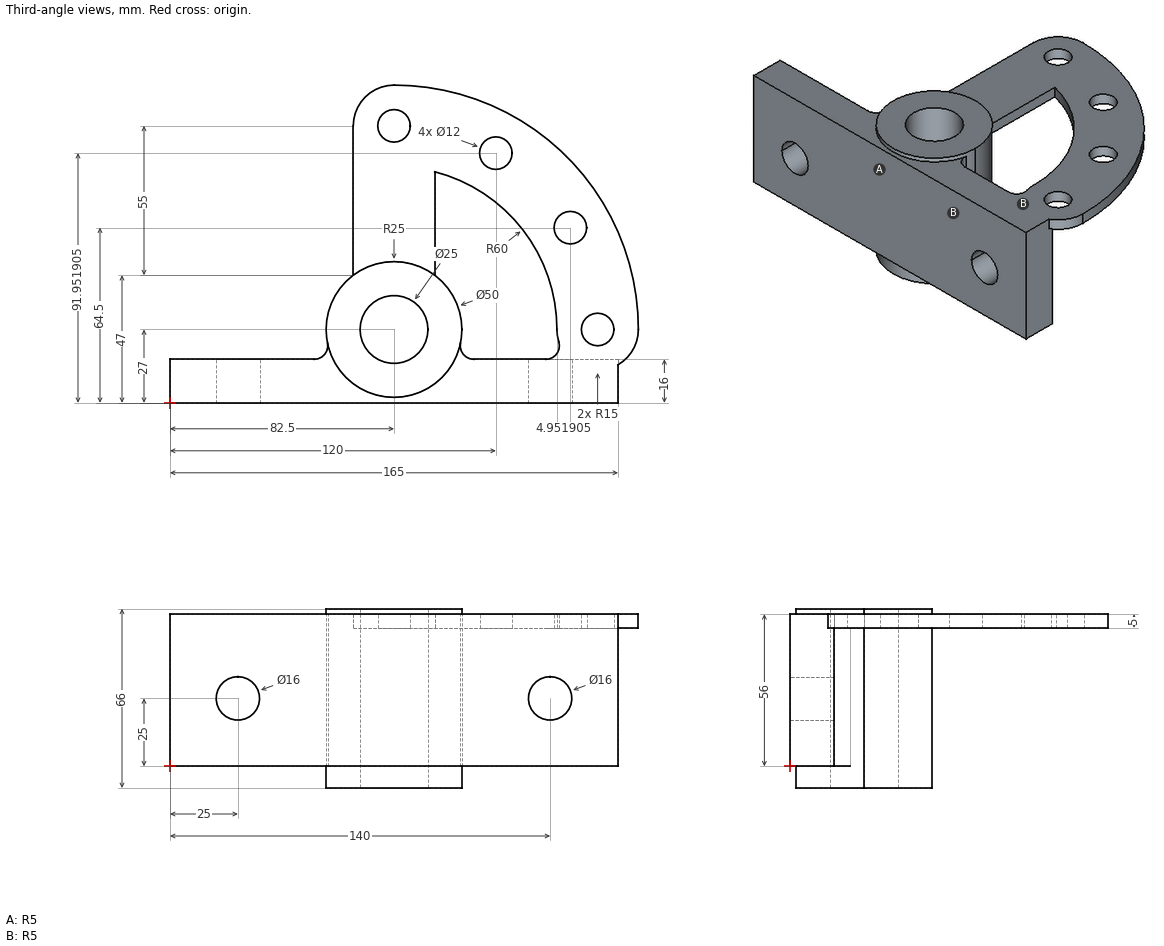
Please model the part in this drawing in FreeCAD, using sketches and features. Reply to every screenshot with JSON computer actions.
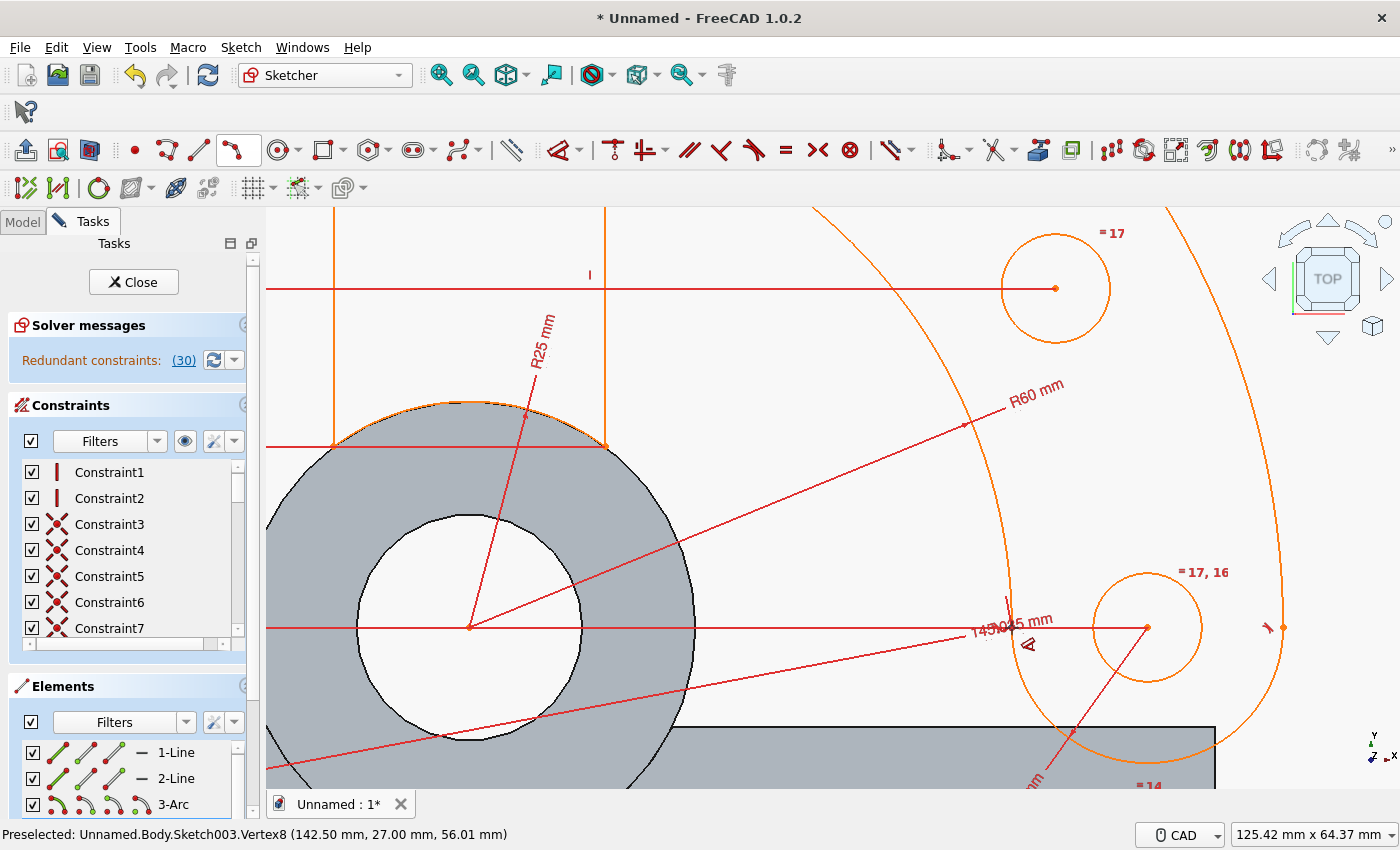
{"action": "left_click", "coordinate": [1056, 289]}
{"action": "left_click", "coordinate": [1034, 662]}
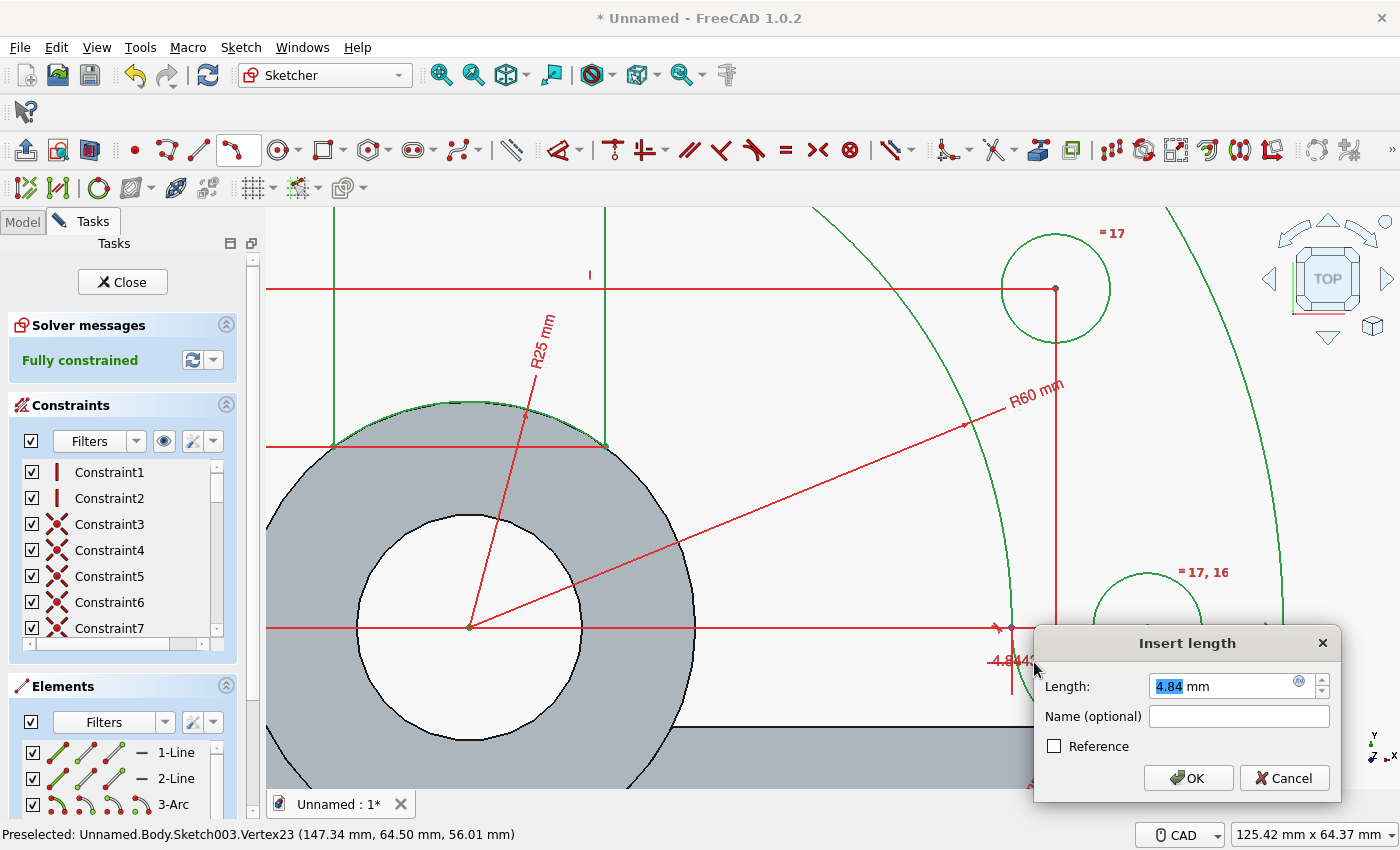
{"action": "type", "text": "4.951905"}
{"action": "key", "text": "Return"}
{"action": "key", "text": "Escape"}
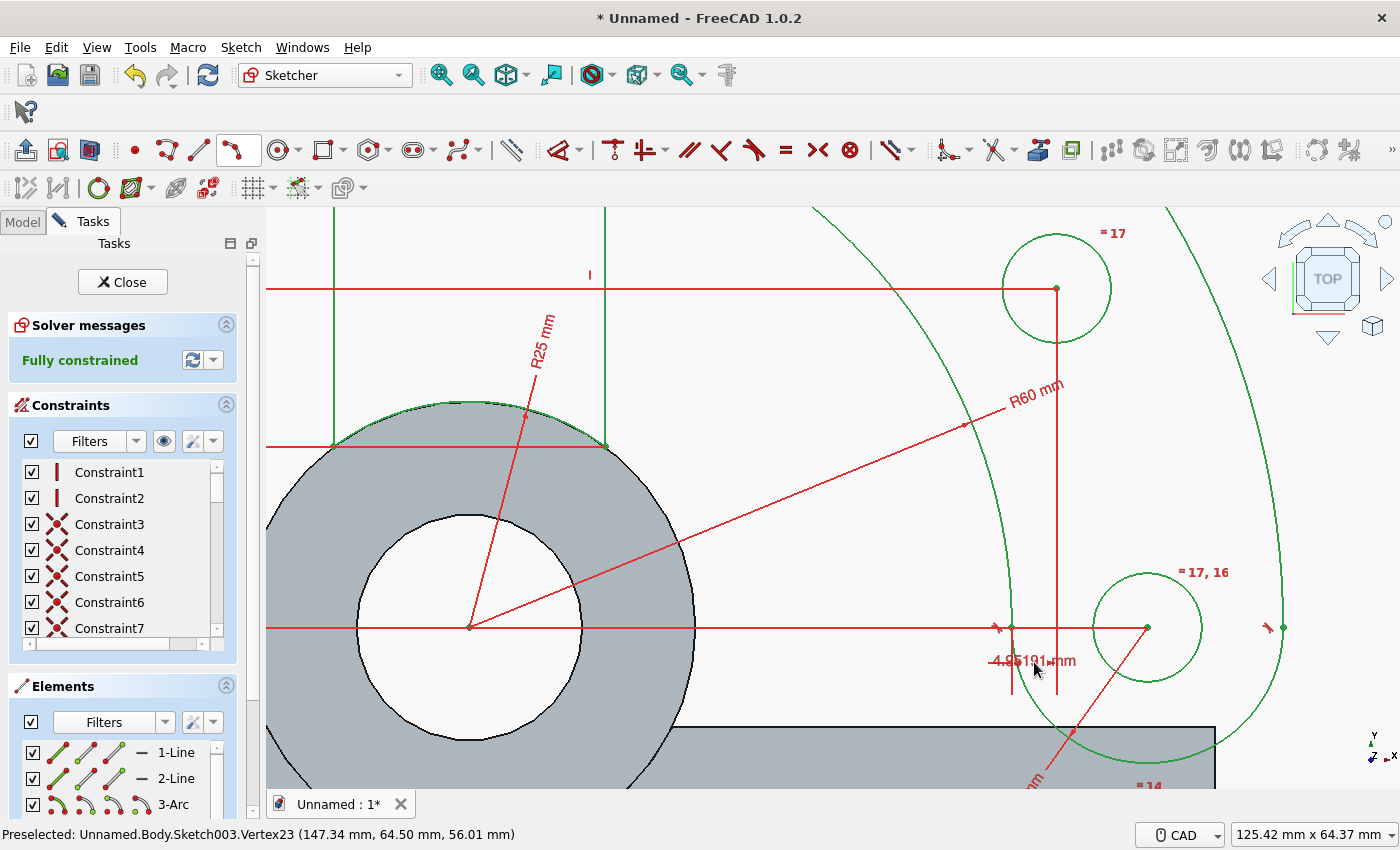
{"action": "left_click", "coordinate": [123, 282]}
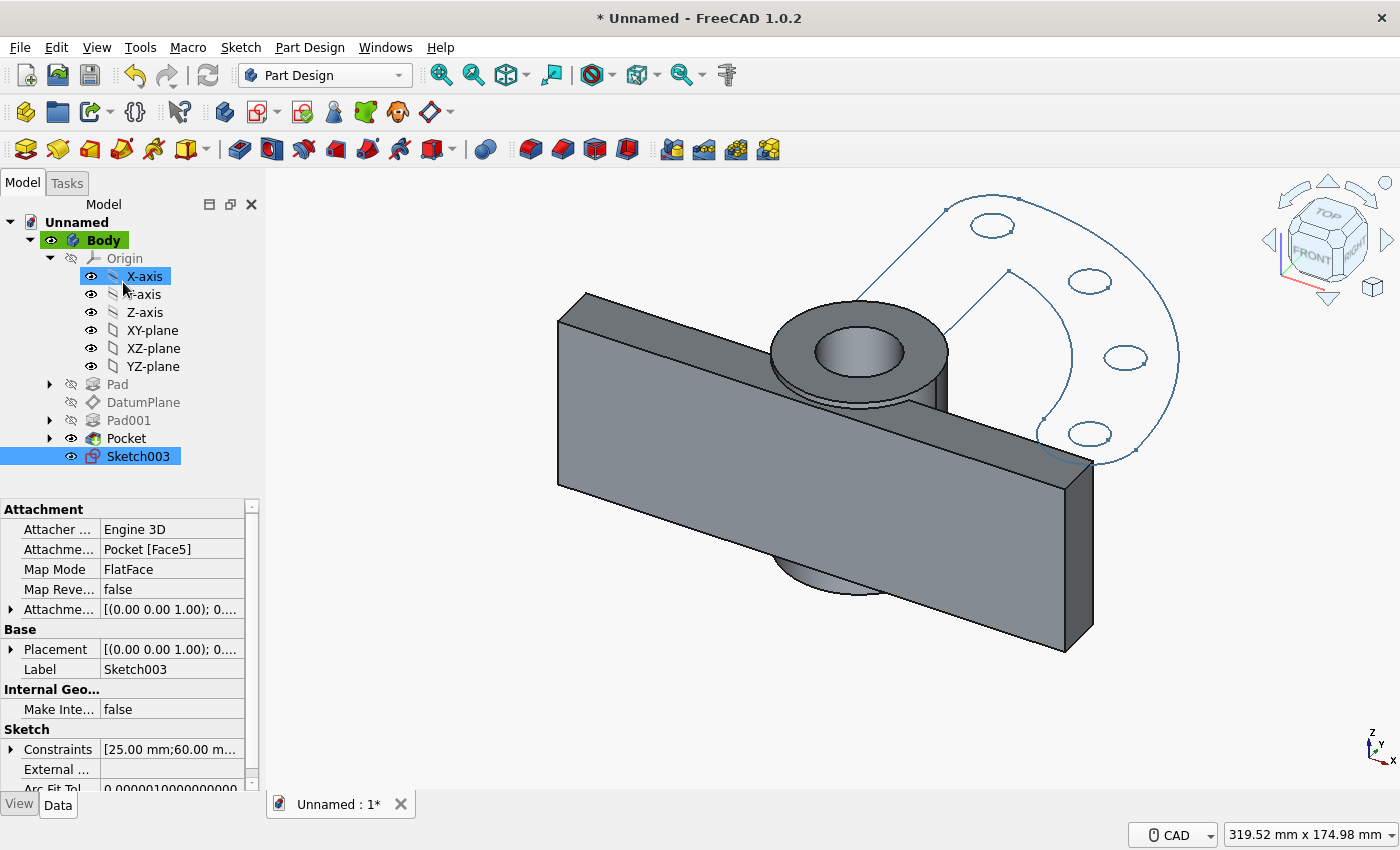
{"action": "left_click", "coordinate": [26, 150]}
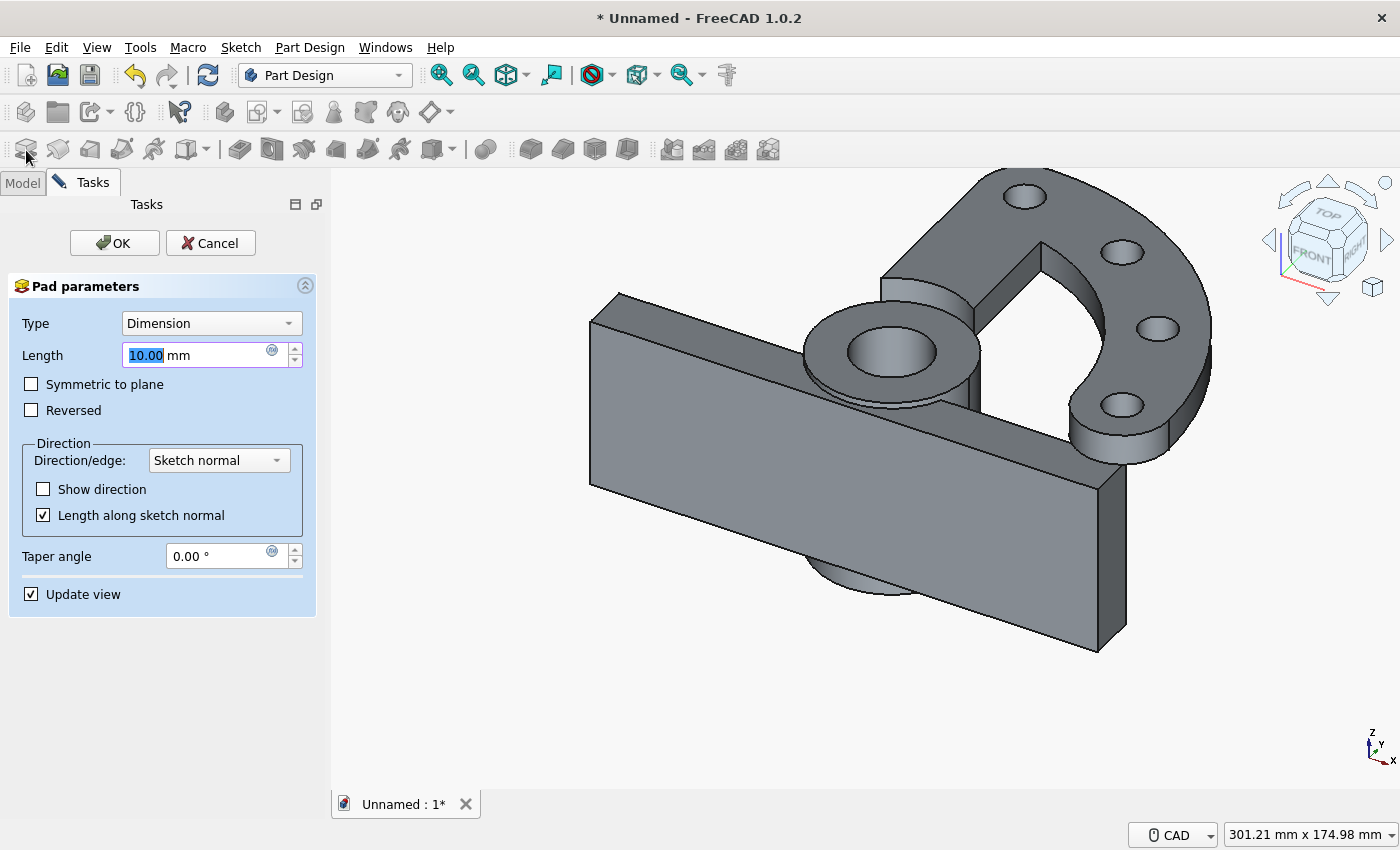
{"action": "type", "text": "5"}
{"action": "key", "text": "Tab"}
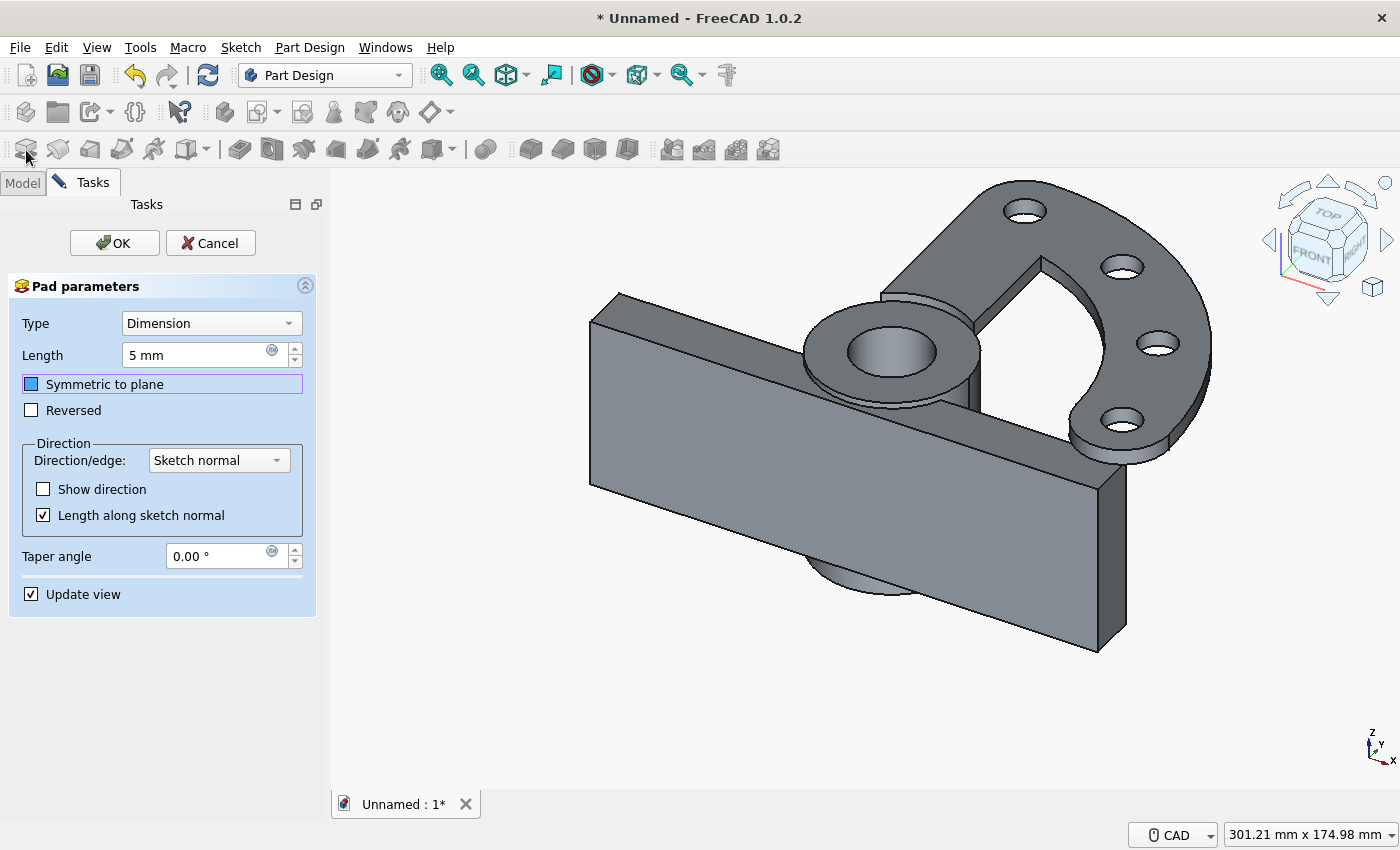
{"action": "left_click", "coordinate": [30, 410]}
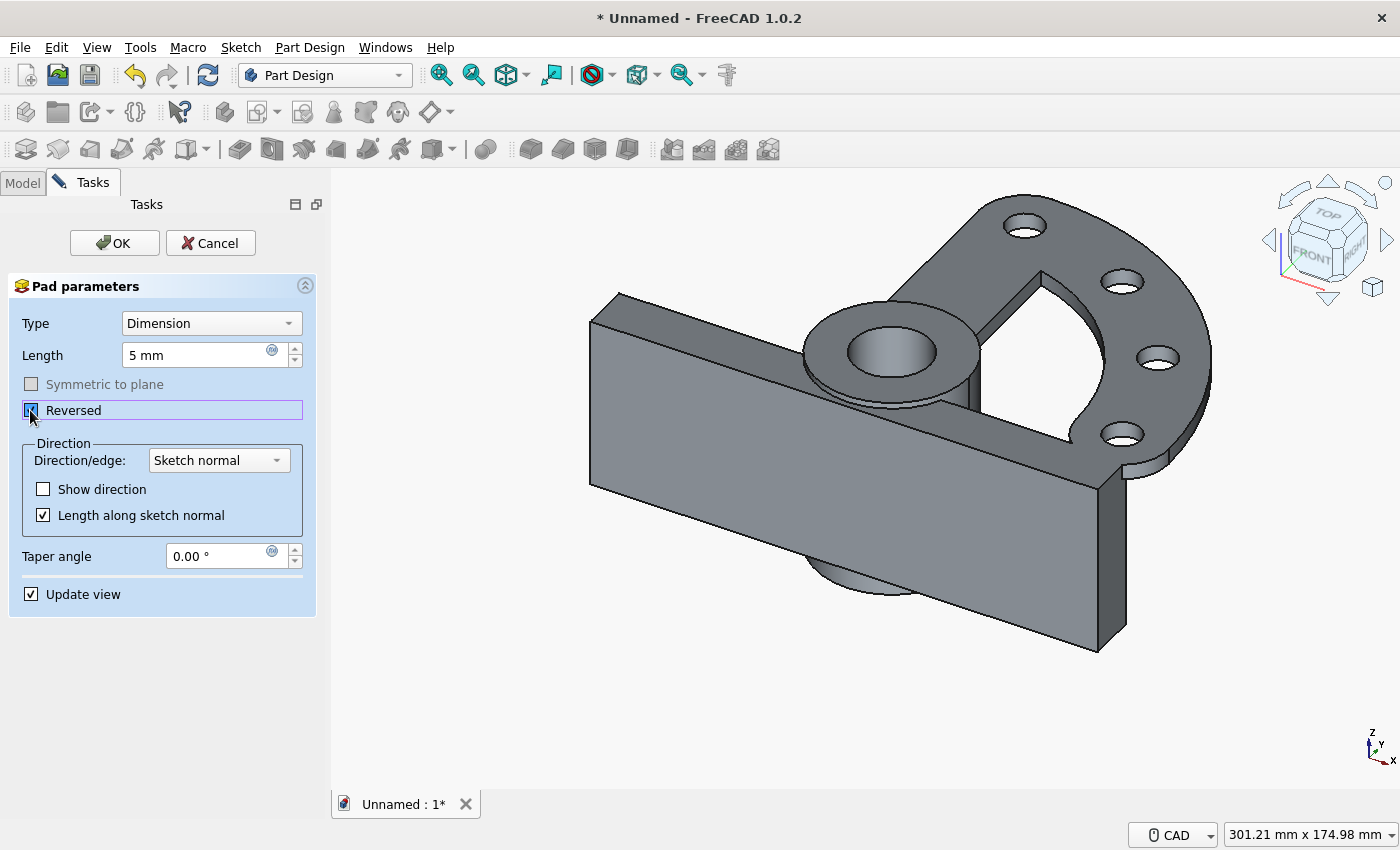
{"action": "left_click", "coordinate": [115, 243]}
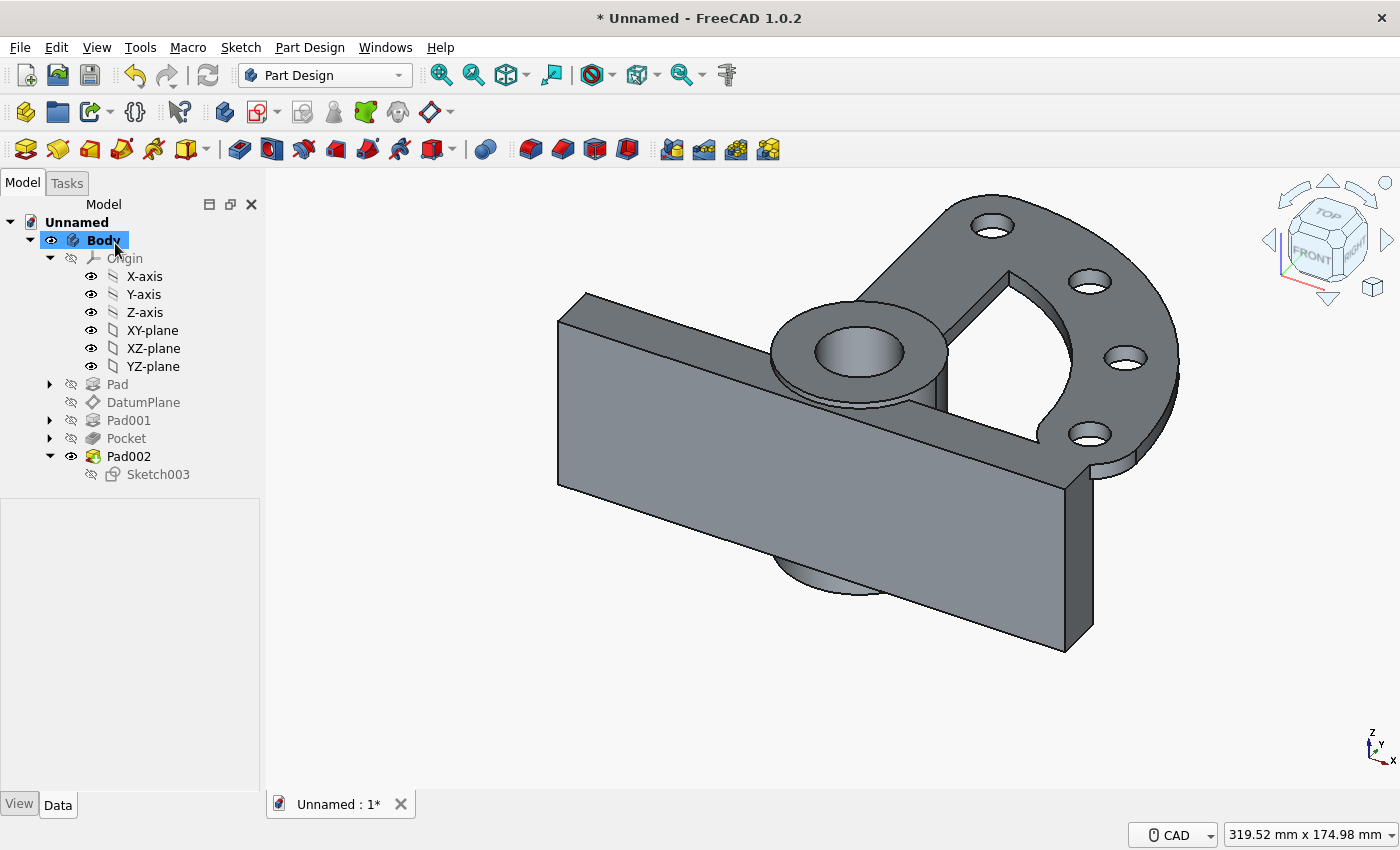
{"action": "left_click", "coordinate": [442, 76]}